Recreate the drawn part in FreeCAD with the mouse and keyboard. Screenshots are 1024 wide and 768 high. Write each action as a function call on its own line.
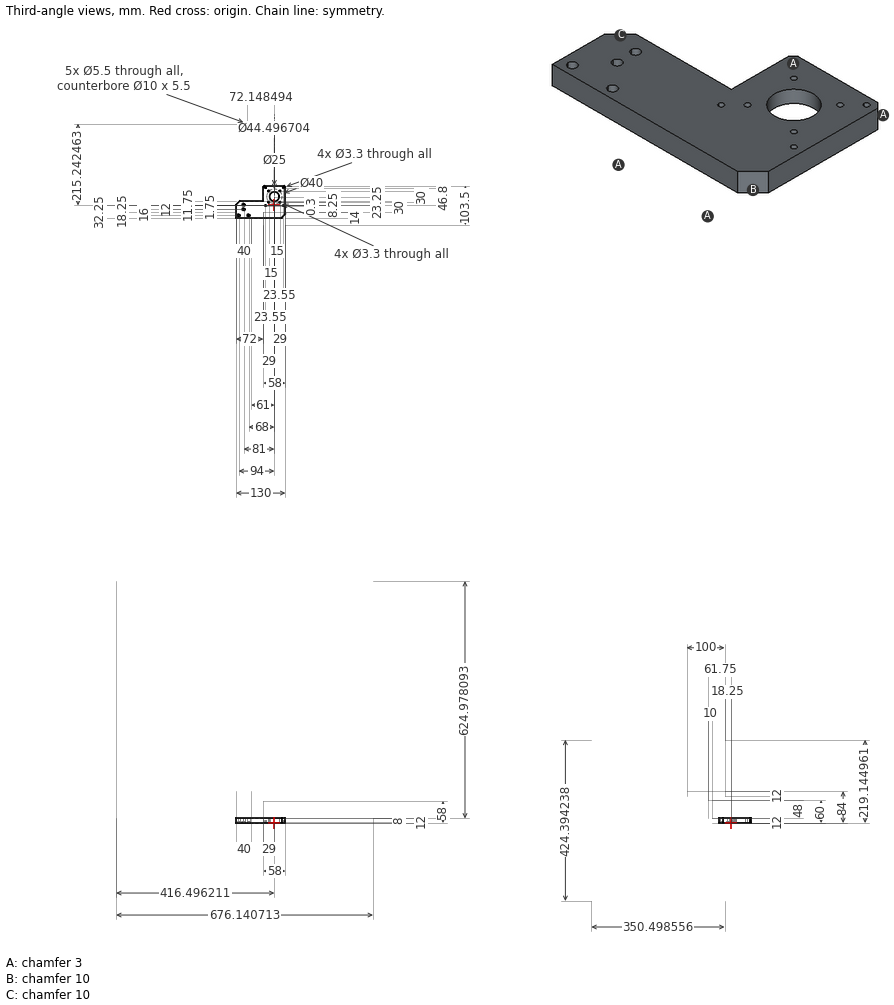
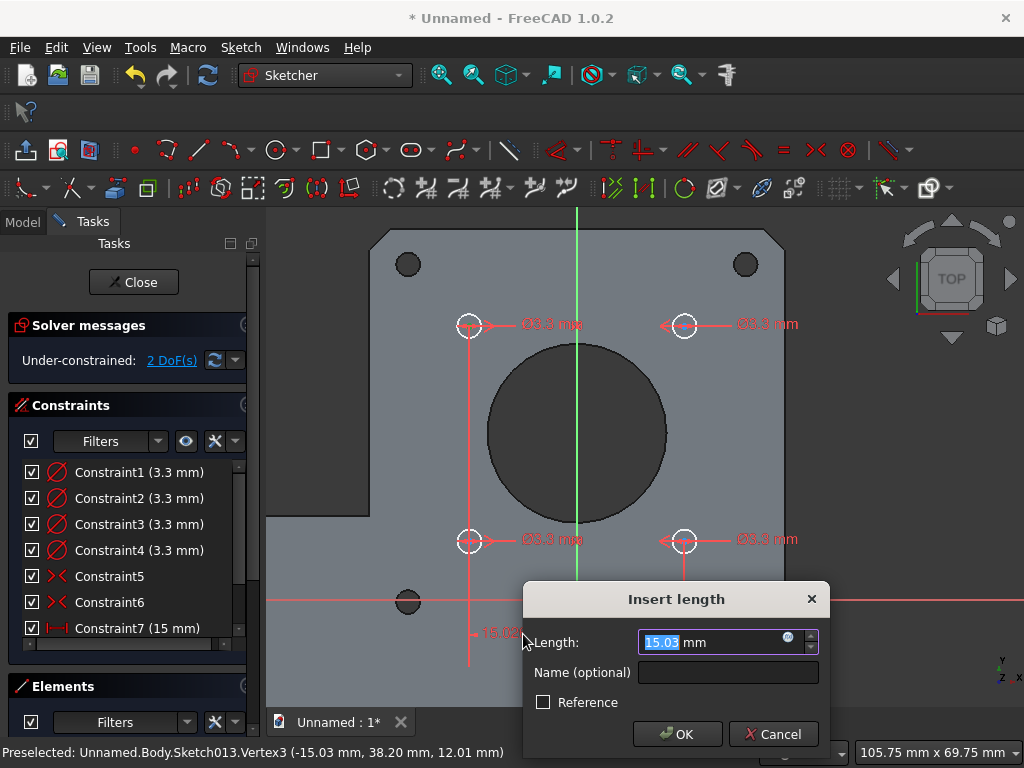
text(15)
key(Return)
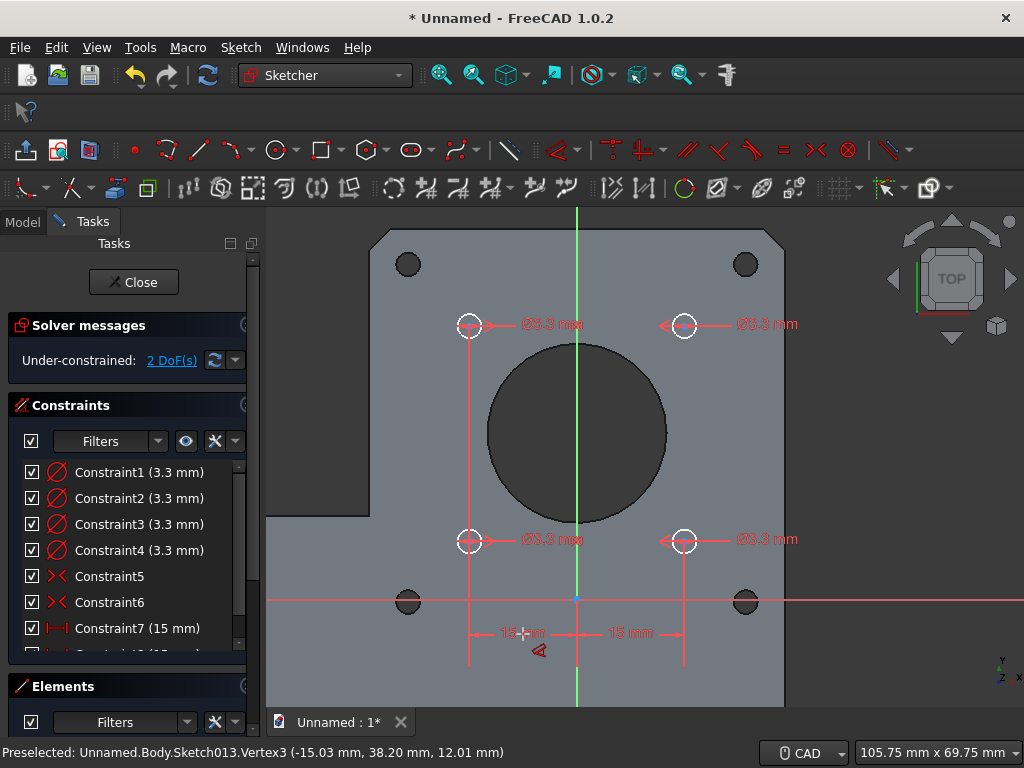
click(469, 541)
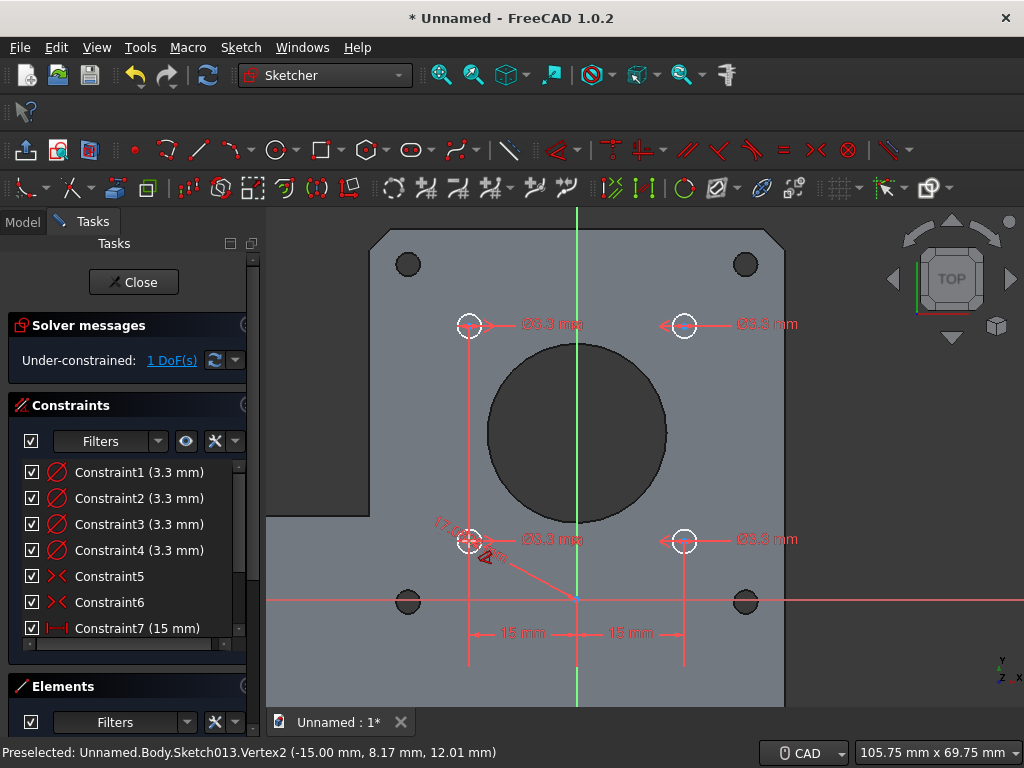
click(469, 326)
click(435, 434)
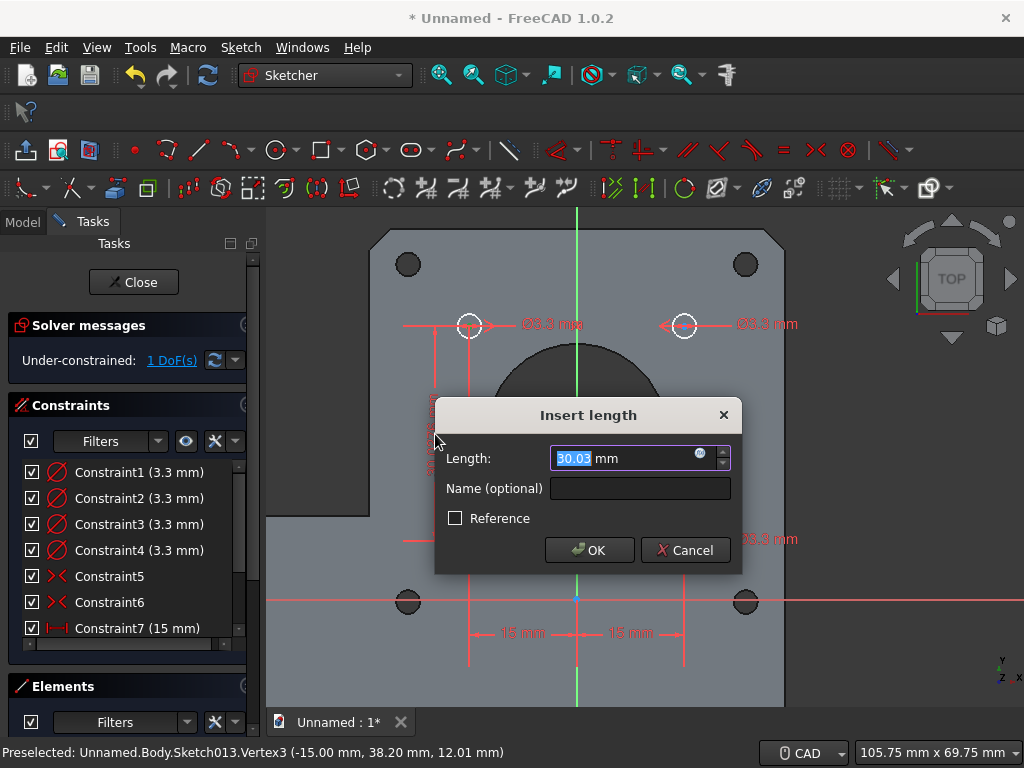
text(30)
key(Return)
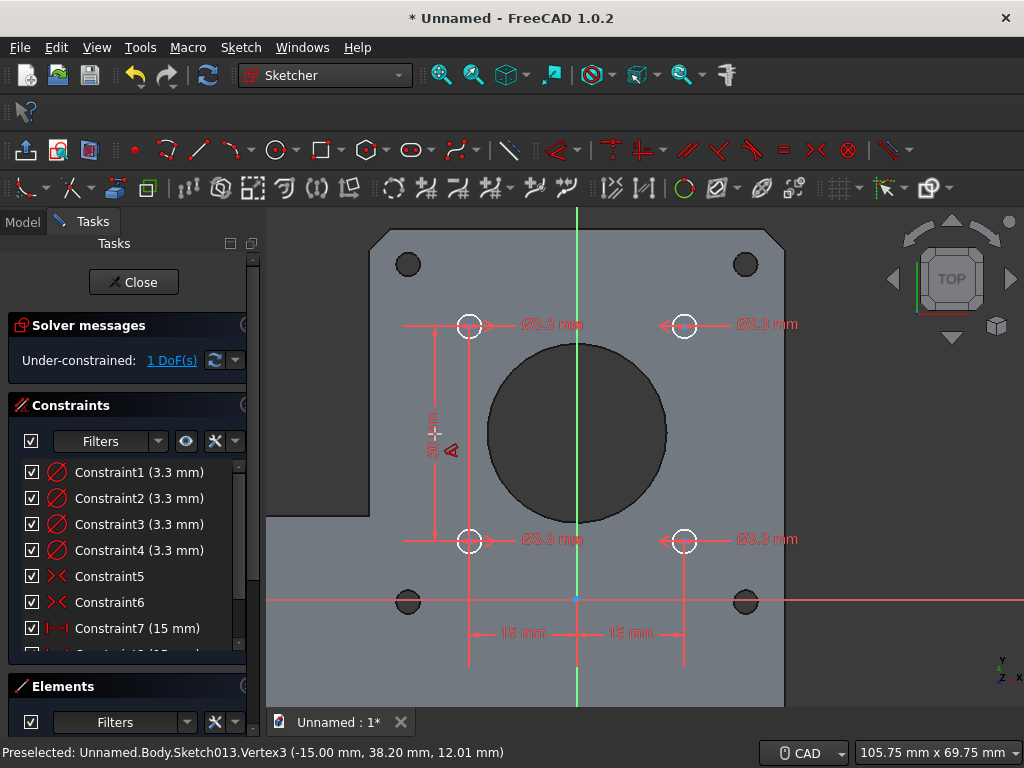
click(684, 541)
click(718, 571)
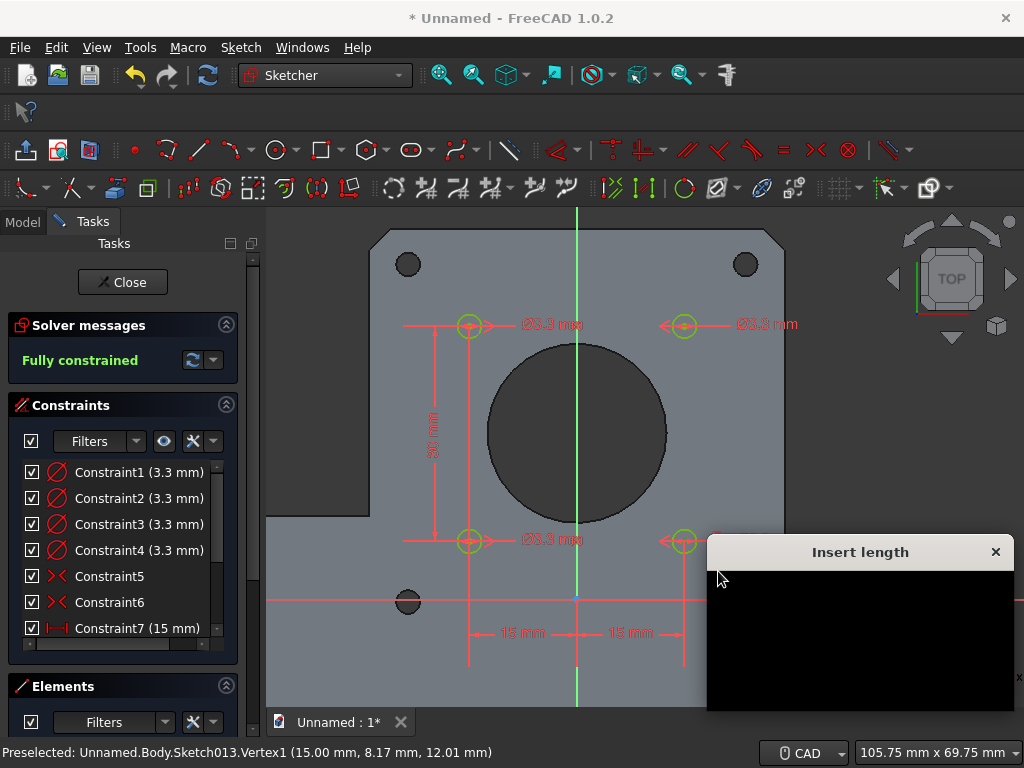
text(8.25)
key(Return)
key(Escape)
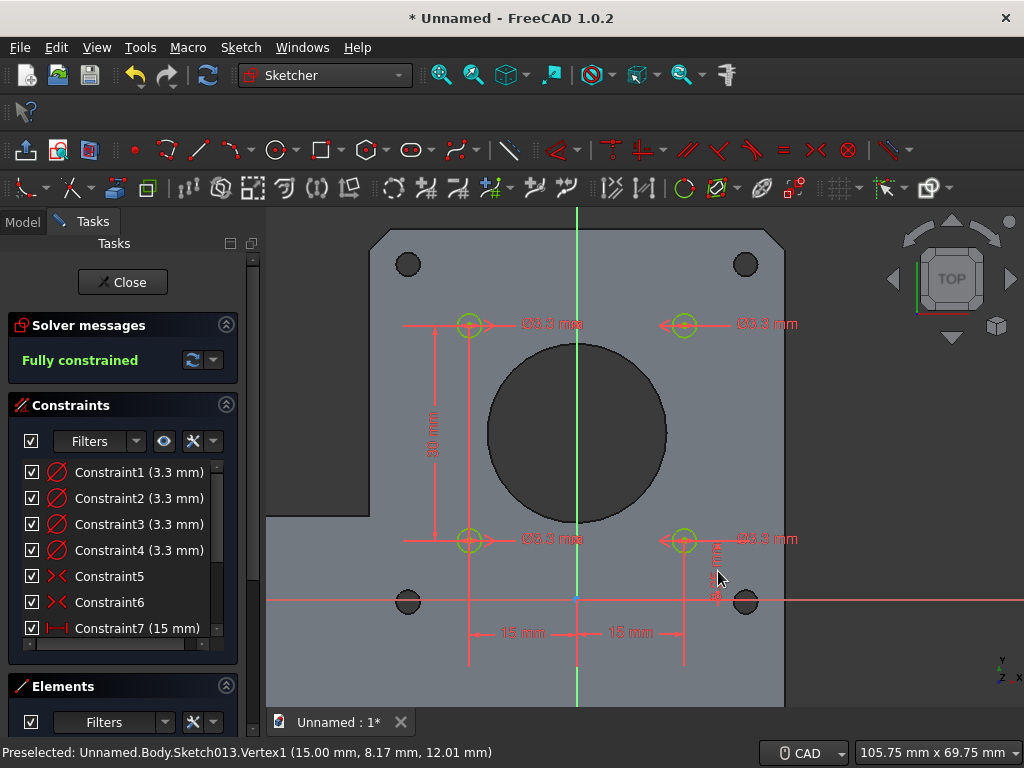
click(123, 282)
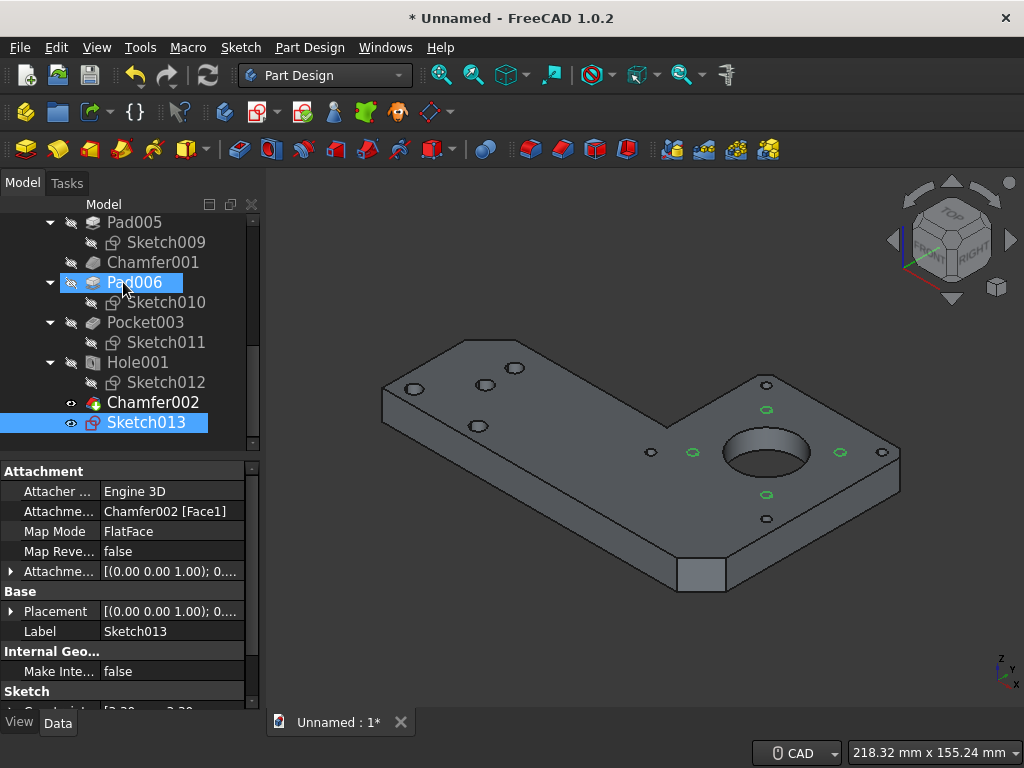
click(272, 150)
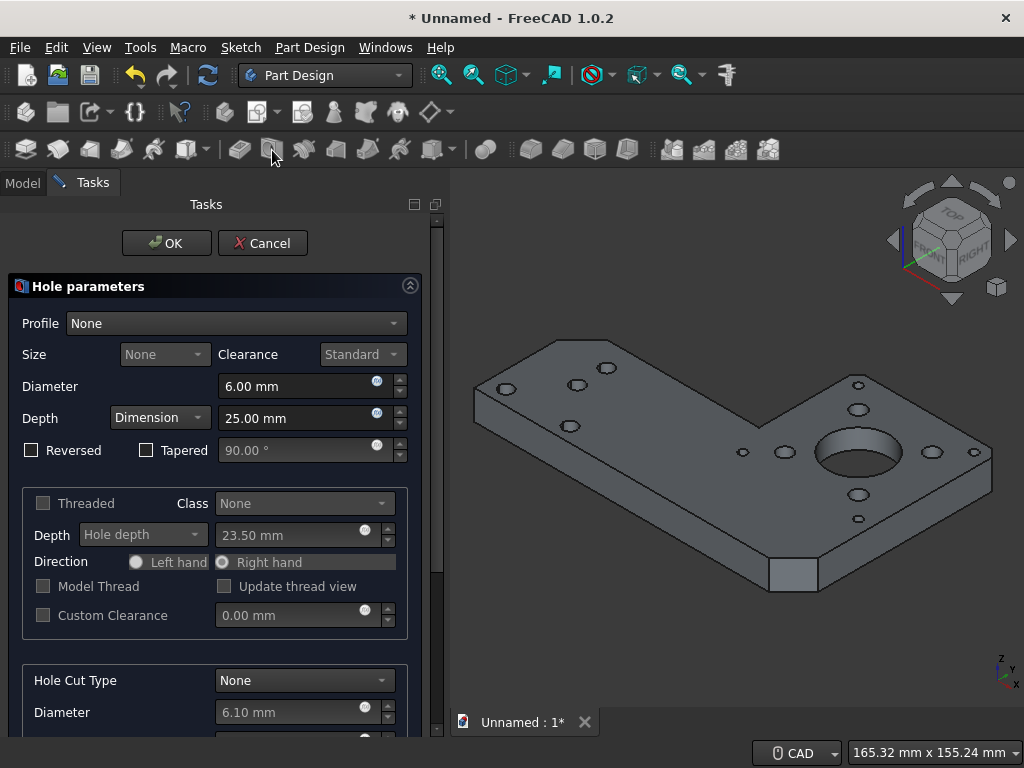
triple_click(305, 386)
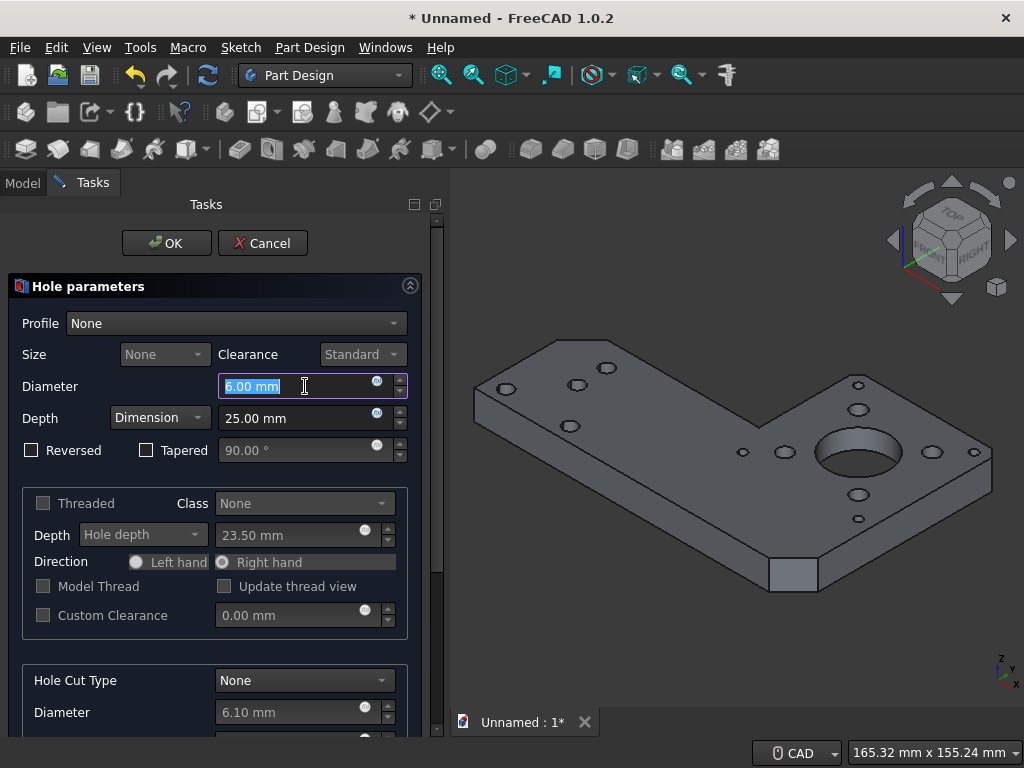
text(3.3)
key(Tab)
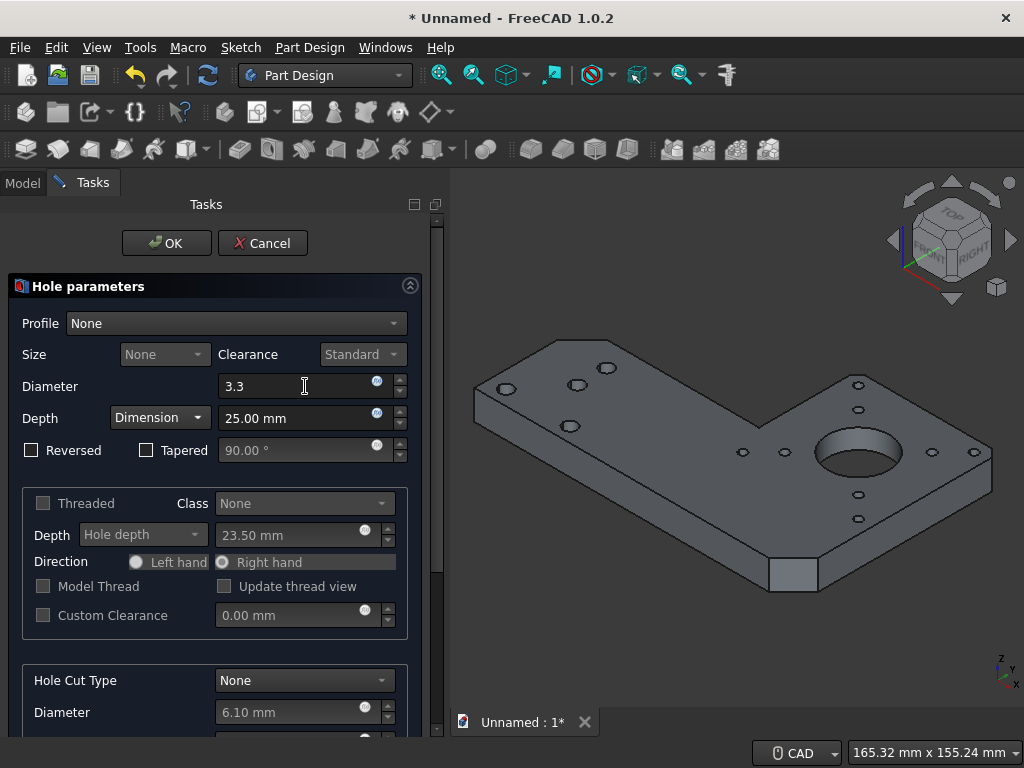
click(161, 418)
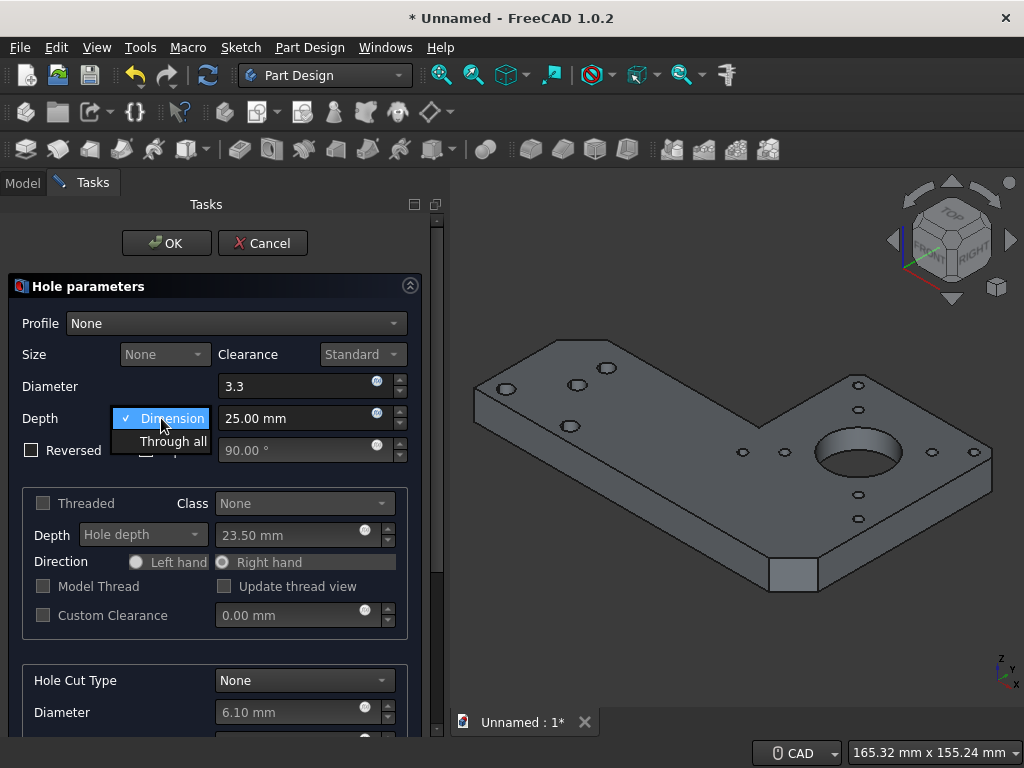
click(160, 442)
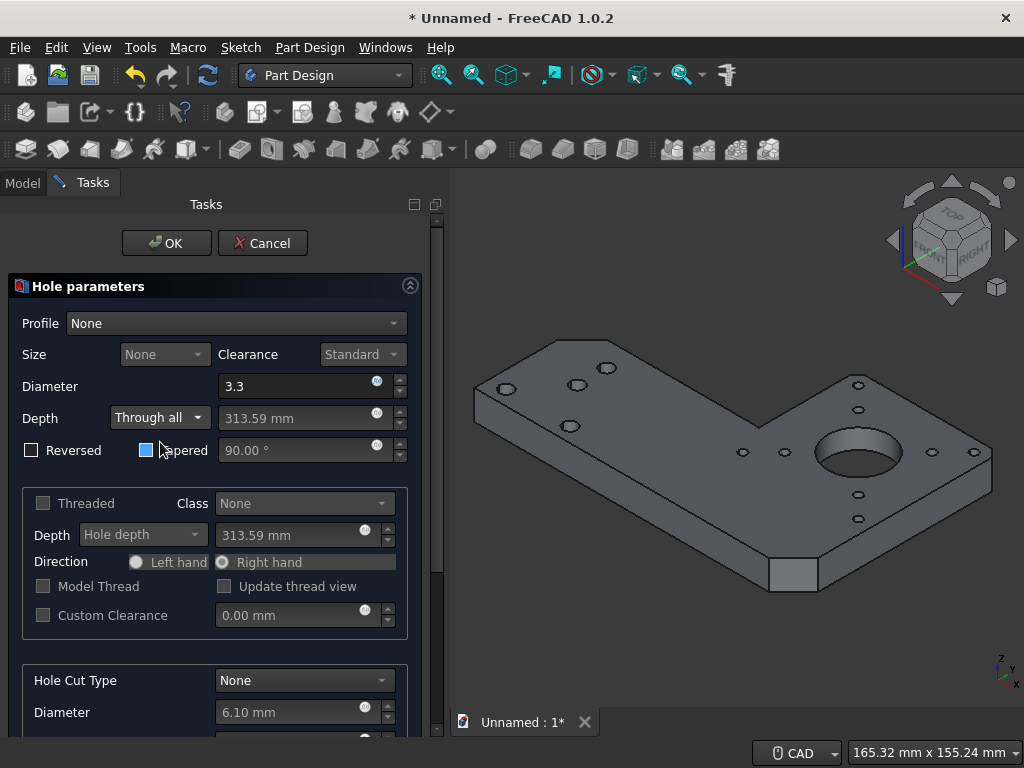
click(167, 243)